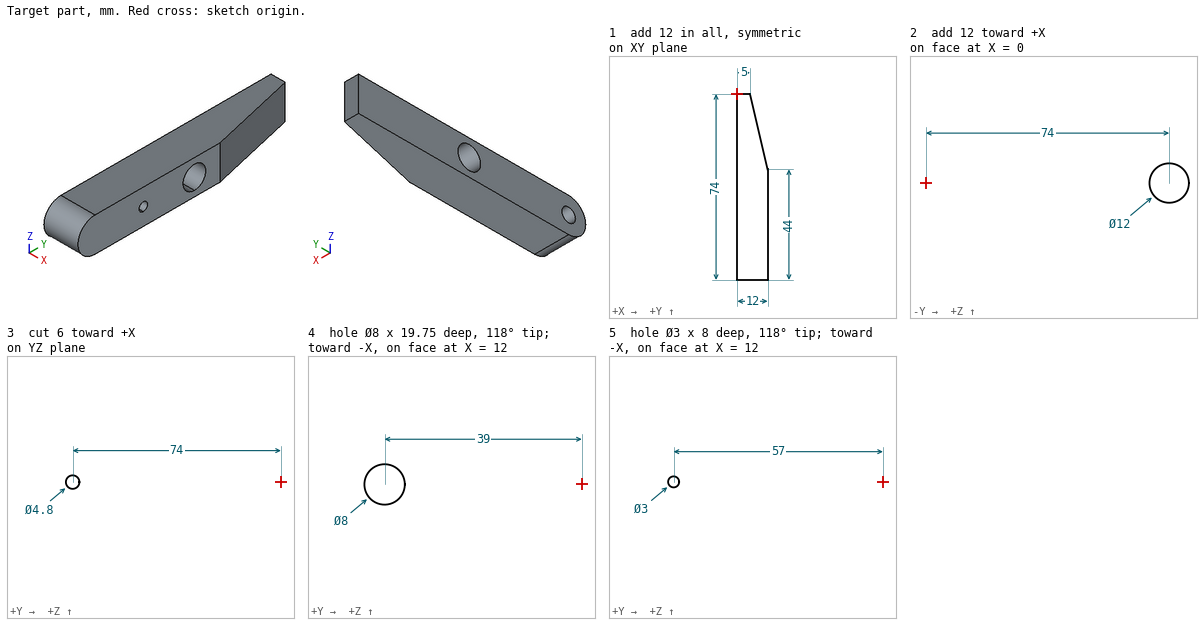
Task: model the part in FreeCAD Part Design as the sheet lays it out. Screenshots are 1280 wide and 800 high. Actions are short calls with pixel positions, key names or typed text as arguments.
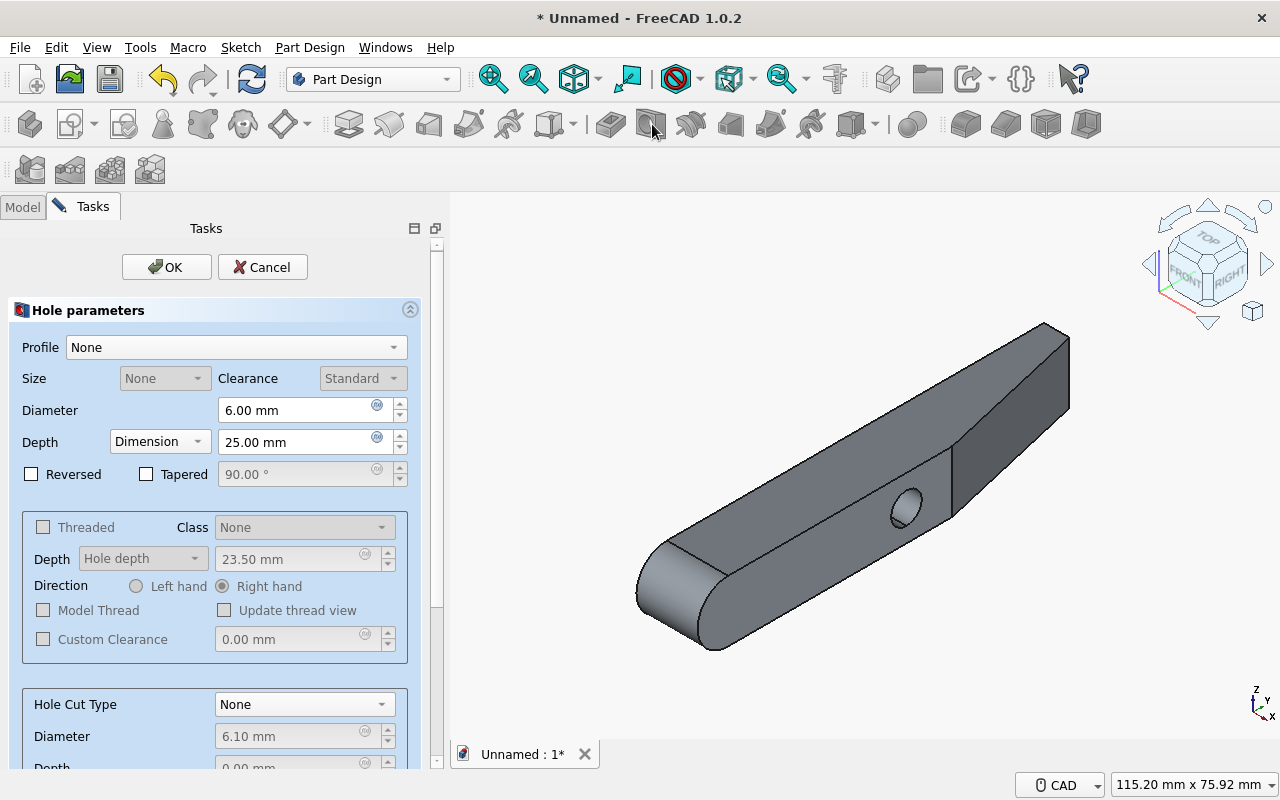
triple_click(305, 410)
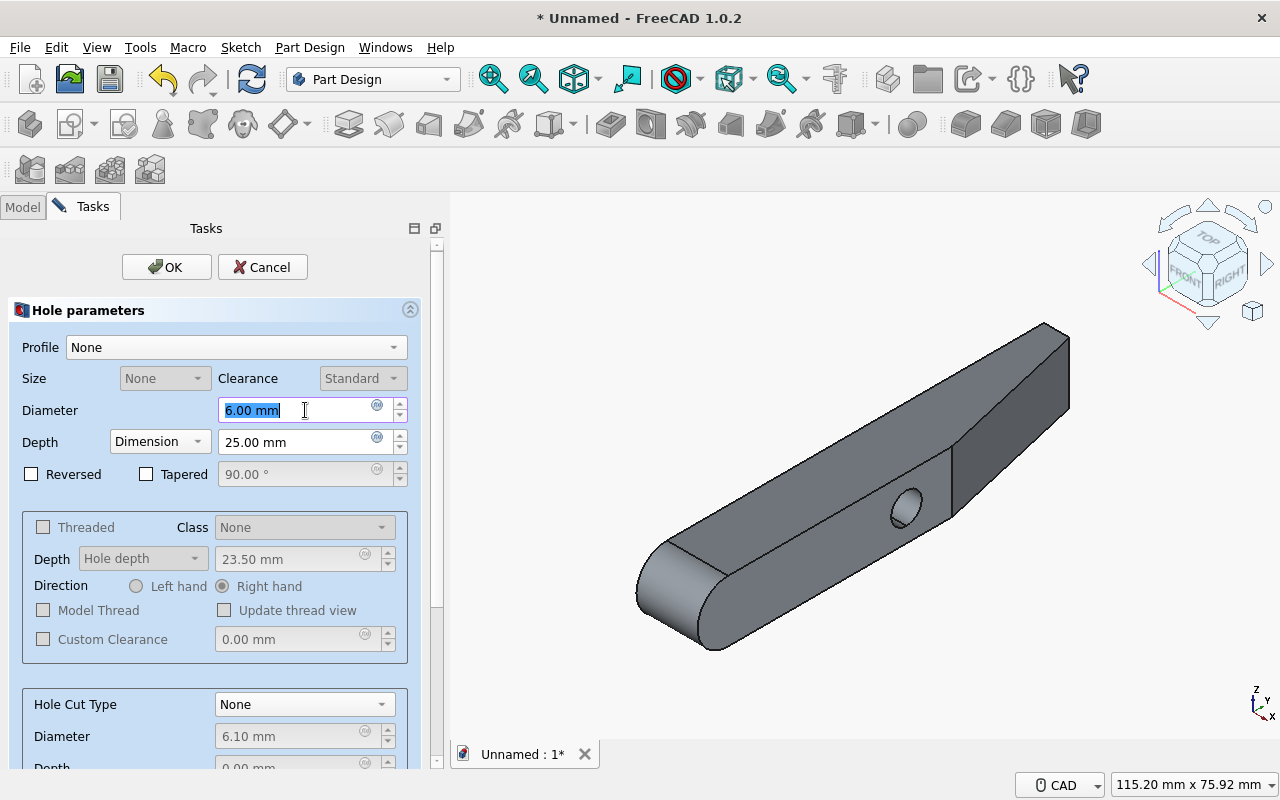
text(8)
key(Tab)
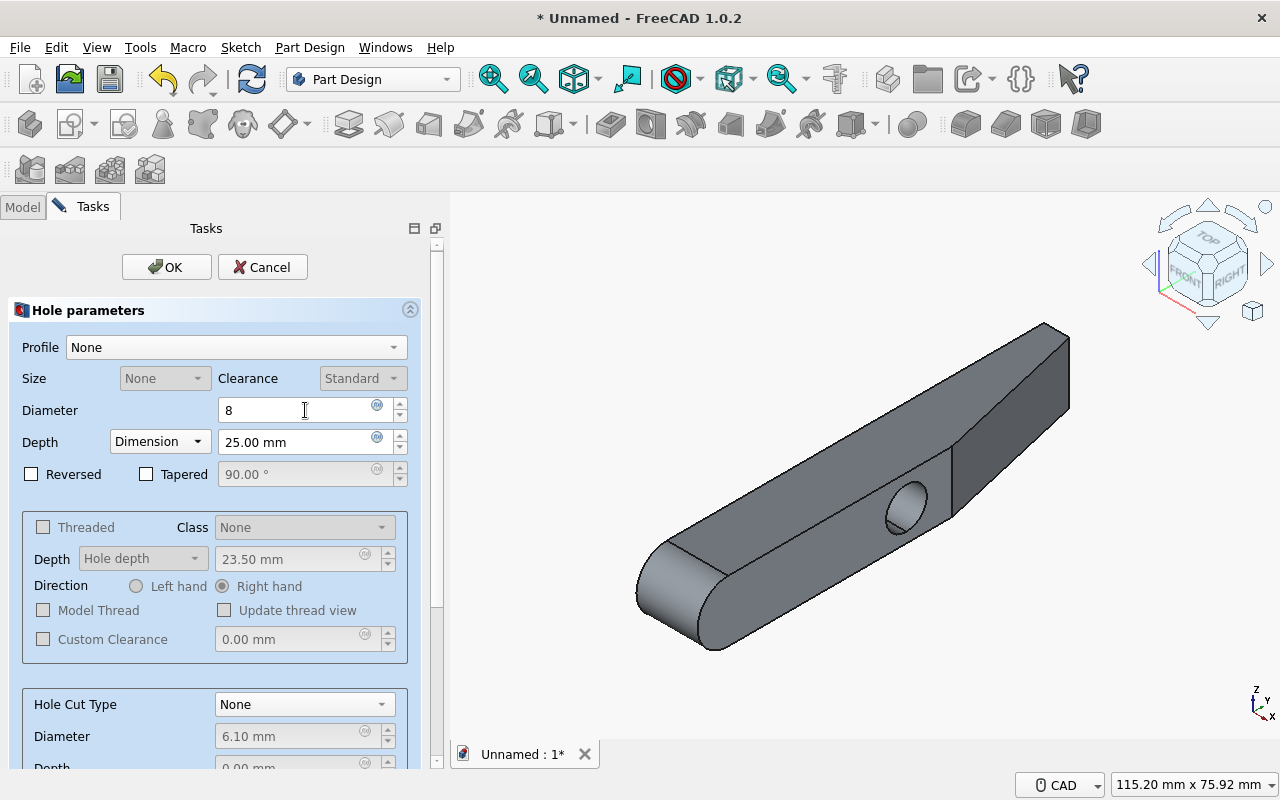
triple_click(305, 442)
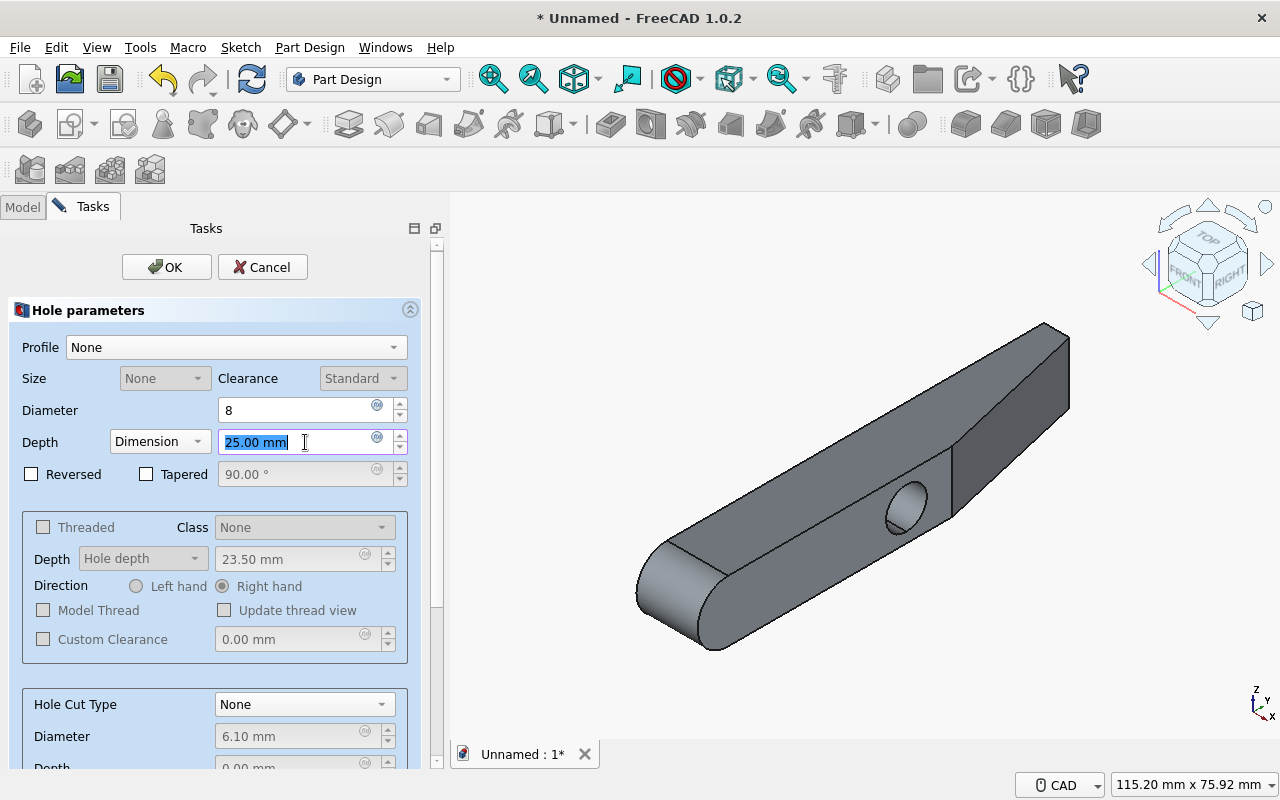
text(19.75)
key(Tab)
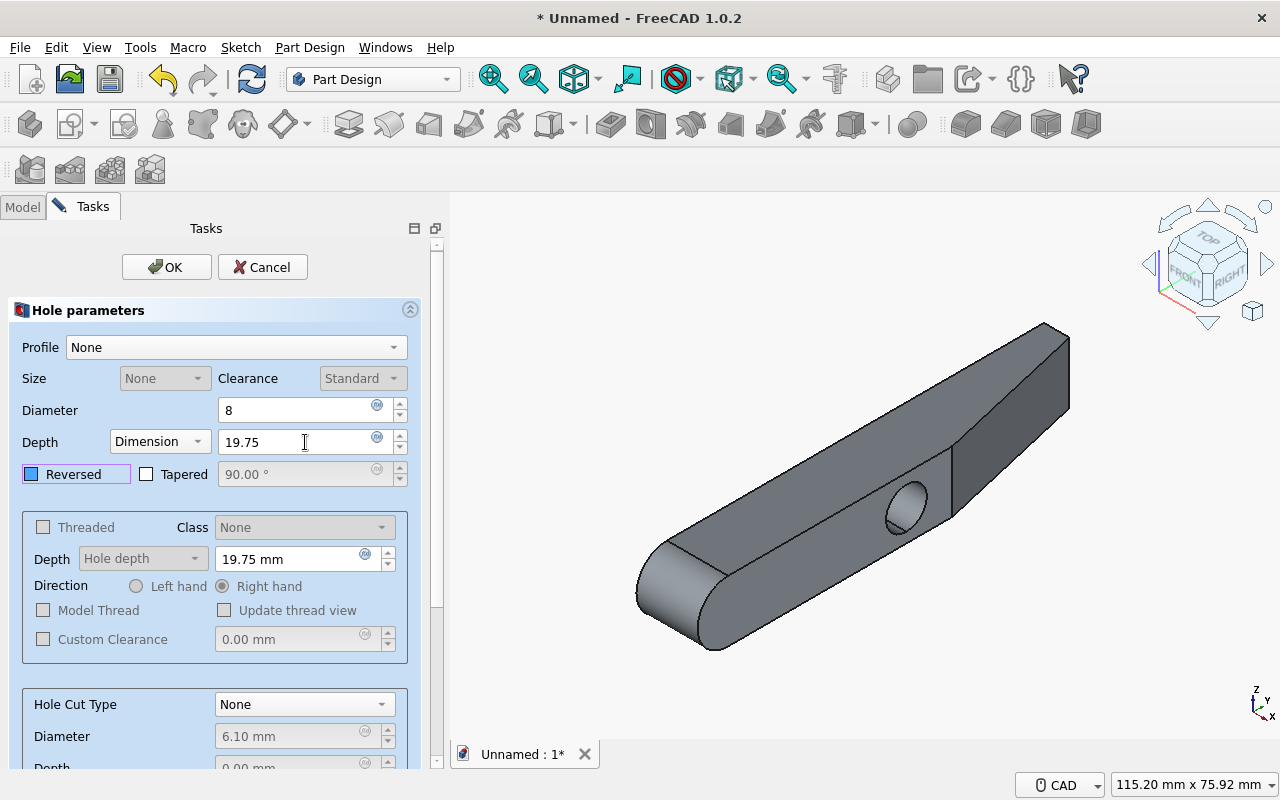
click(167, 267)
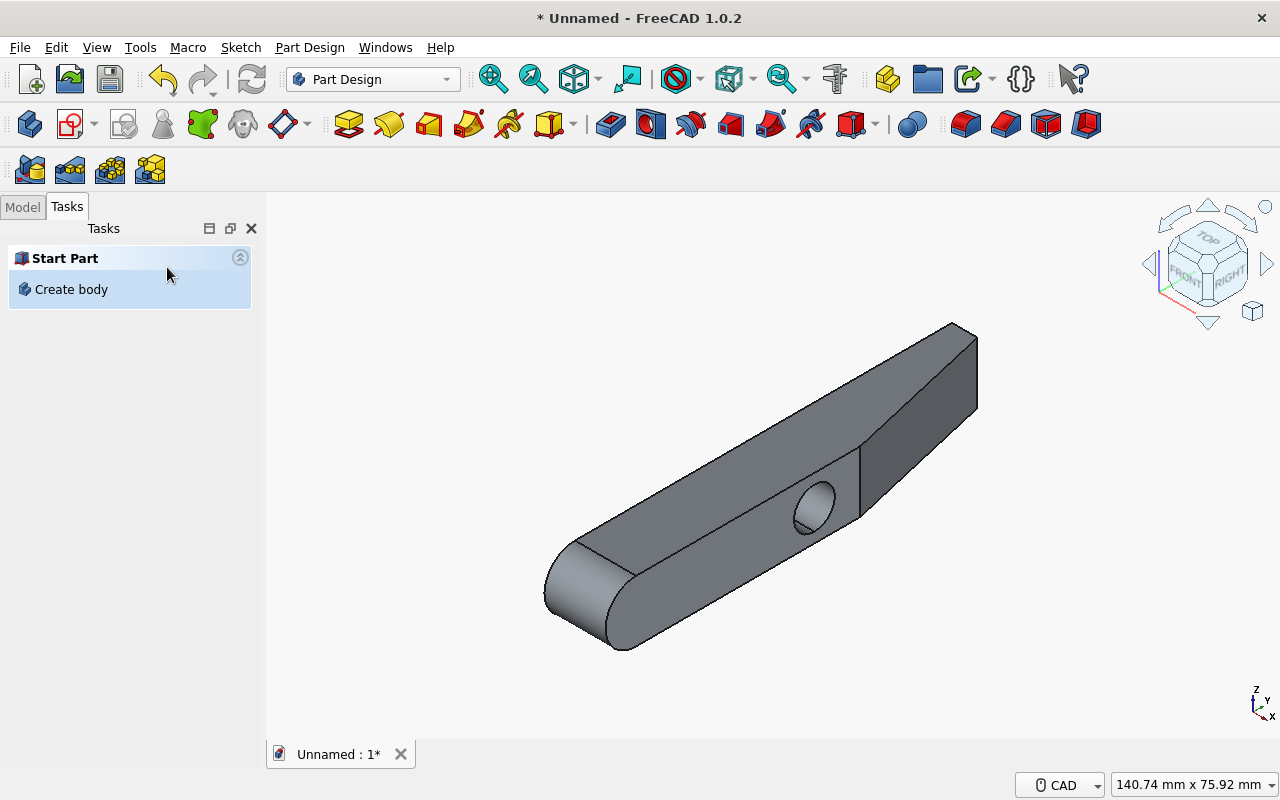
click(733, 554)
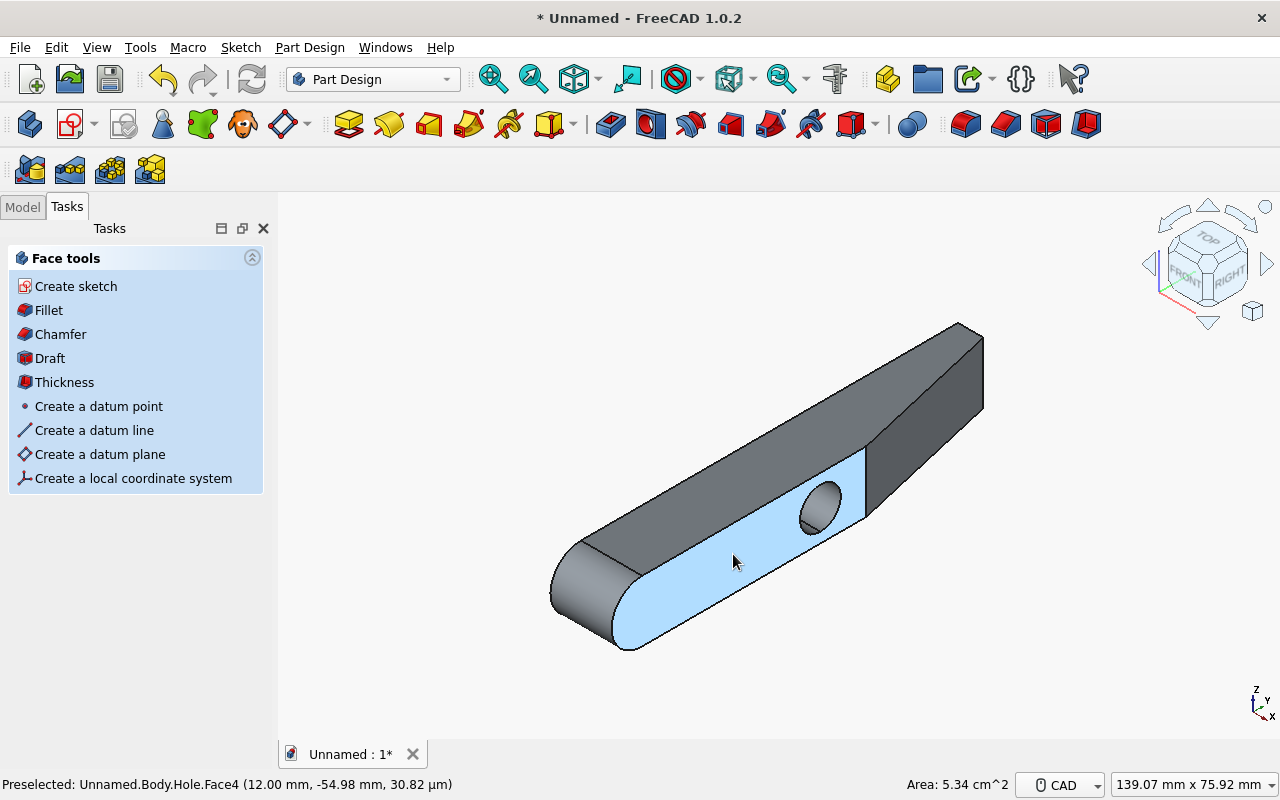
click(70, 124)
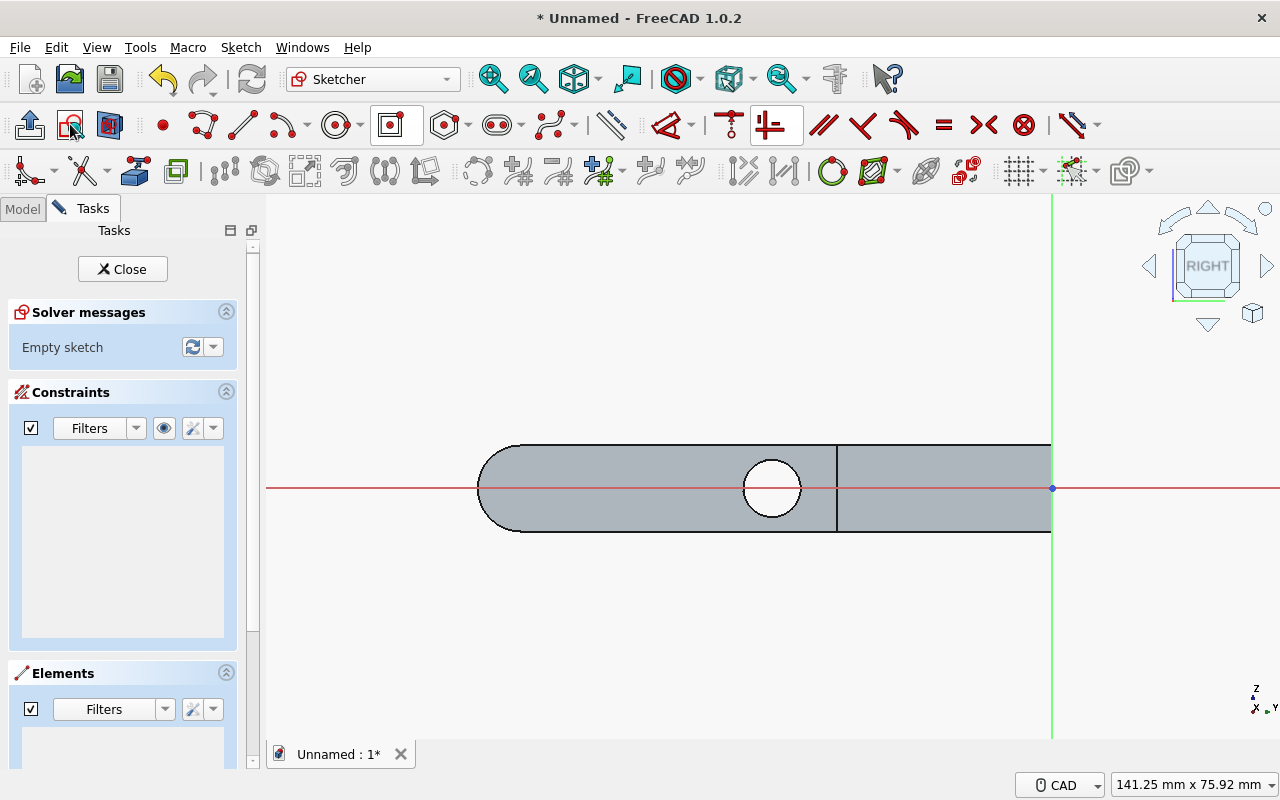
scroll(639, 490, up, 14)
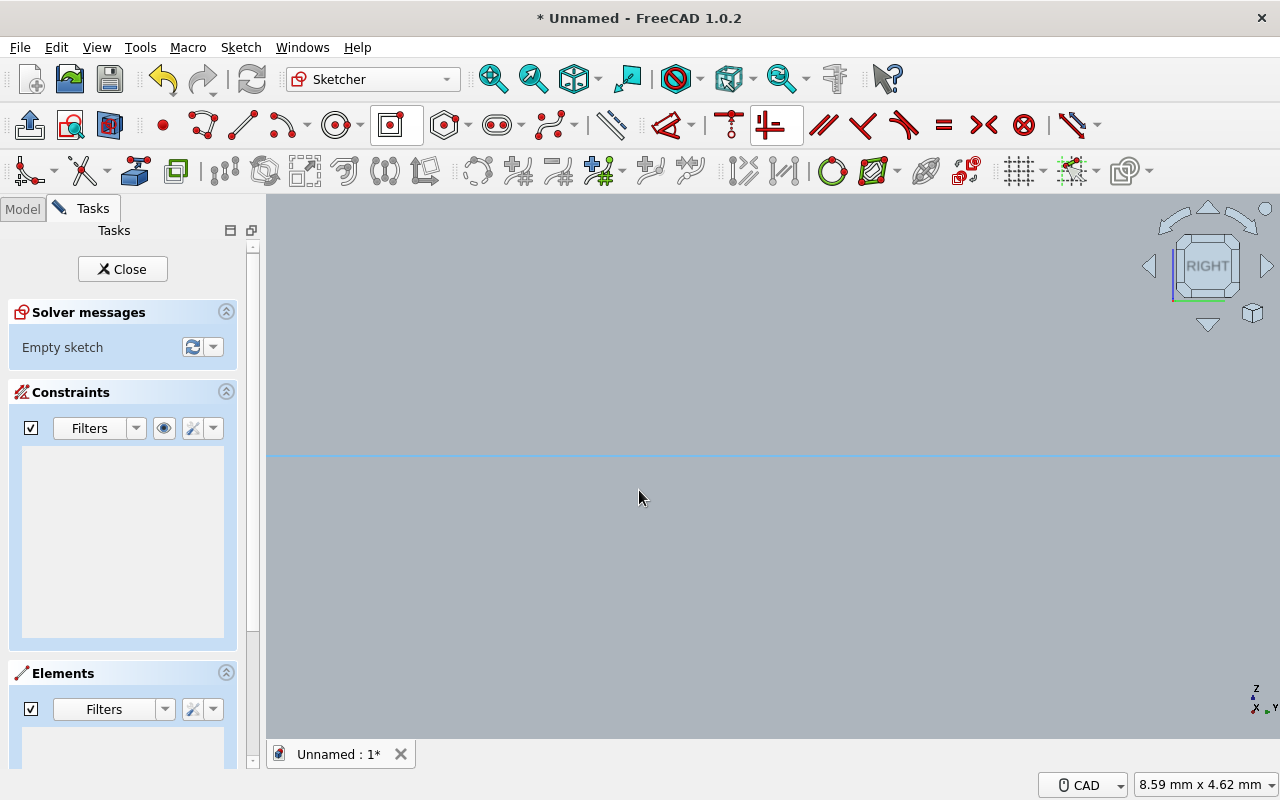
key(g)
key(c)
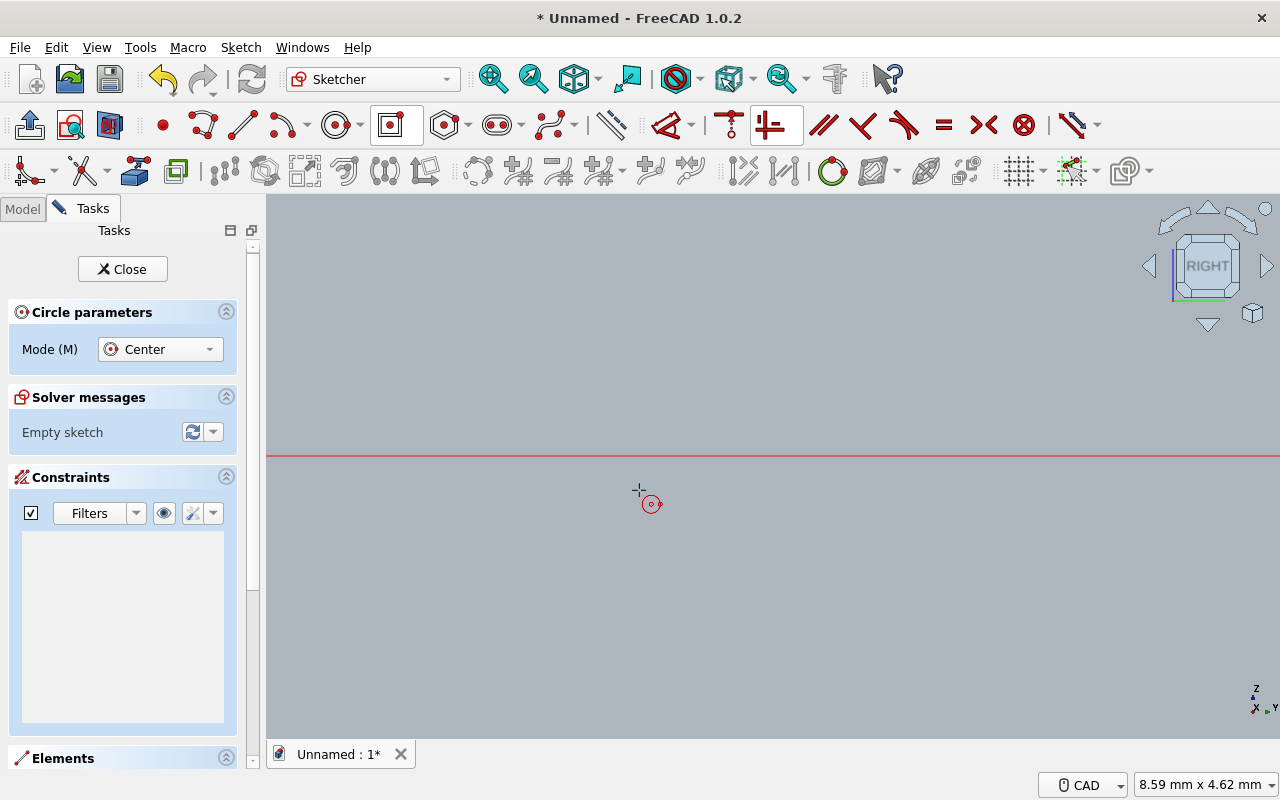
click(697, 456)
move(822, 331)